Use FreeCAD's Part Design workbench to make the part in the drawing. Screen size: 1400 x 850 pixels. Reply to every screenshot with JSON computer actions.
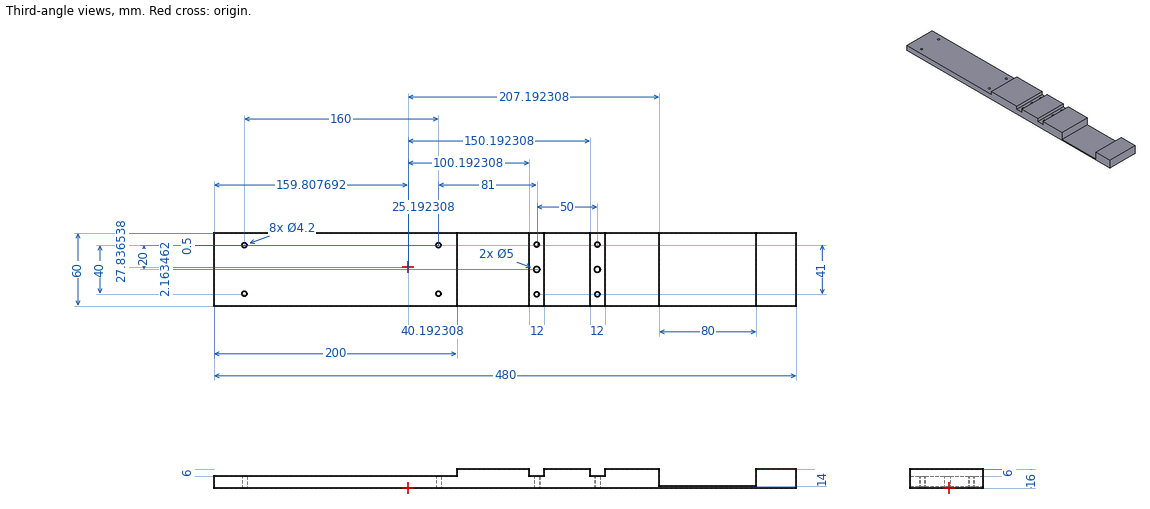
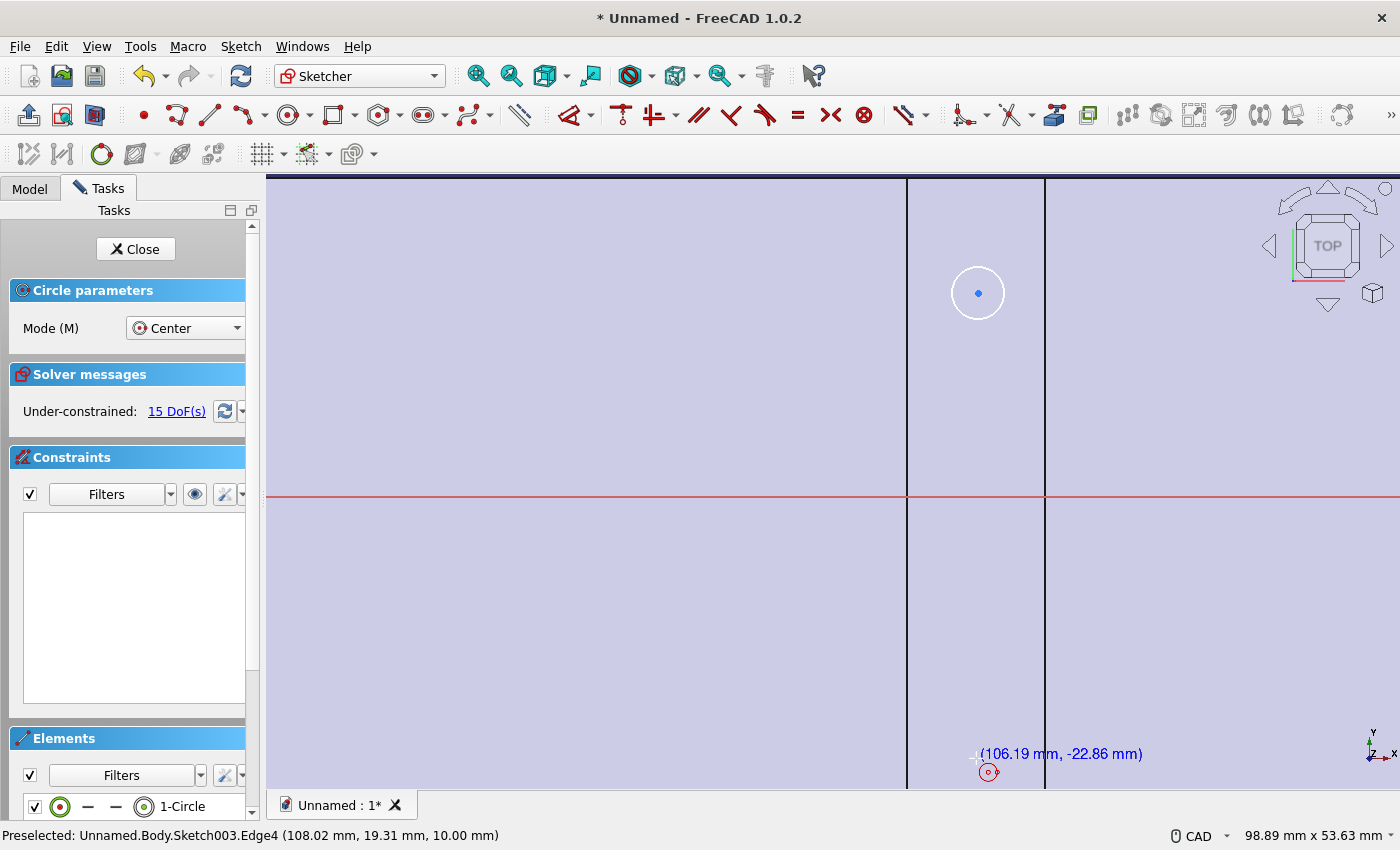
{"action": "scroll", "coordinate": [988, 471], "scroll_direction": "down", "scroll_amount": 8}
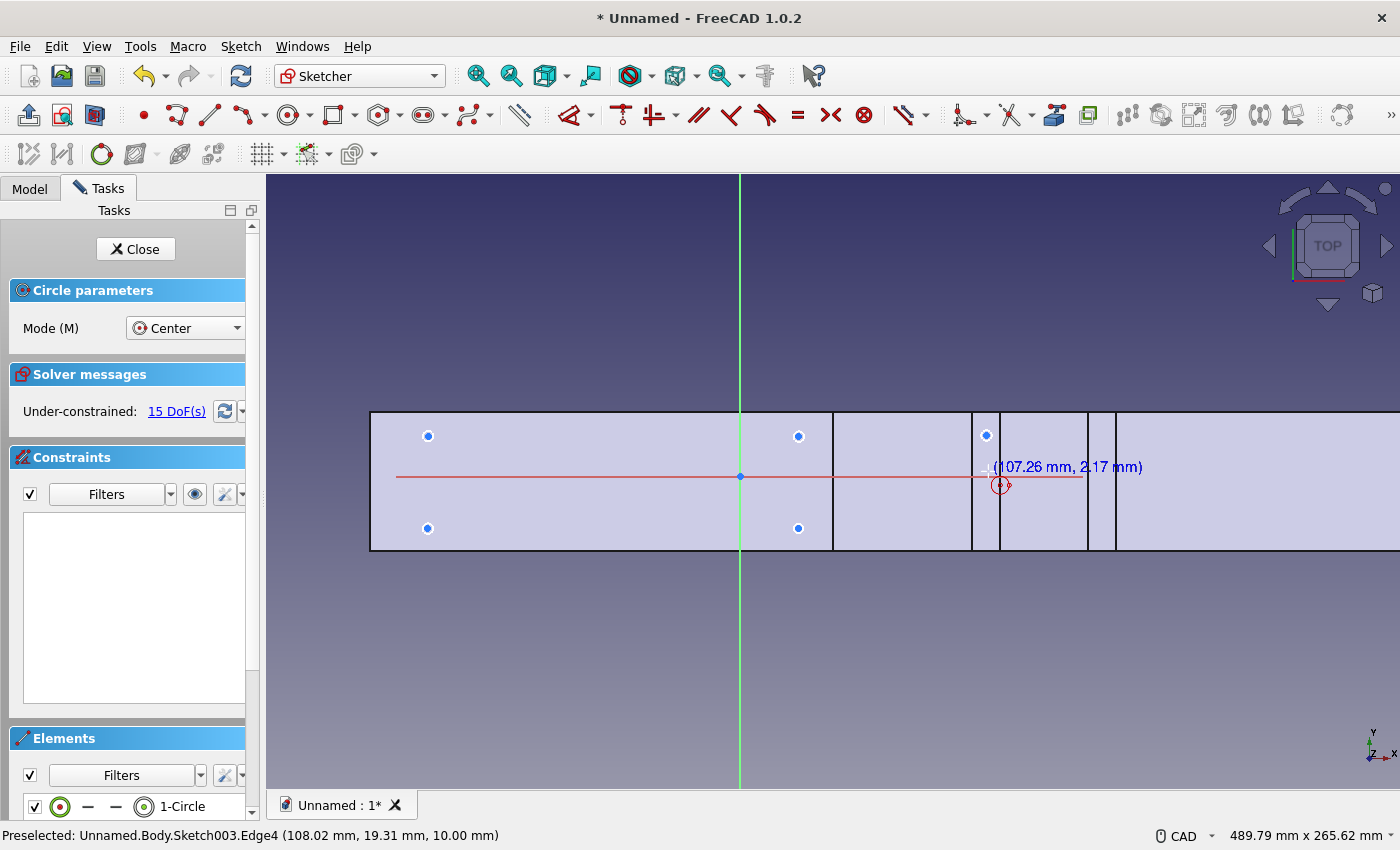
{"action": "left_click", "coordinate": [986, 529]}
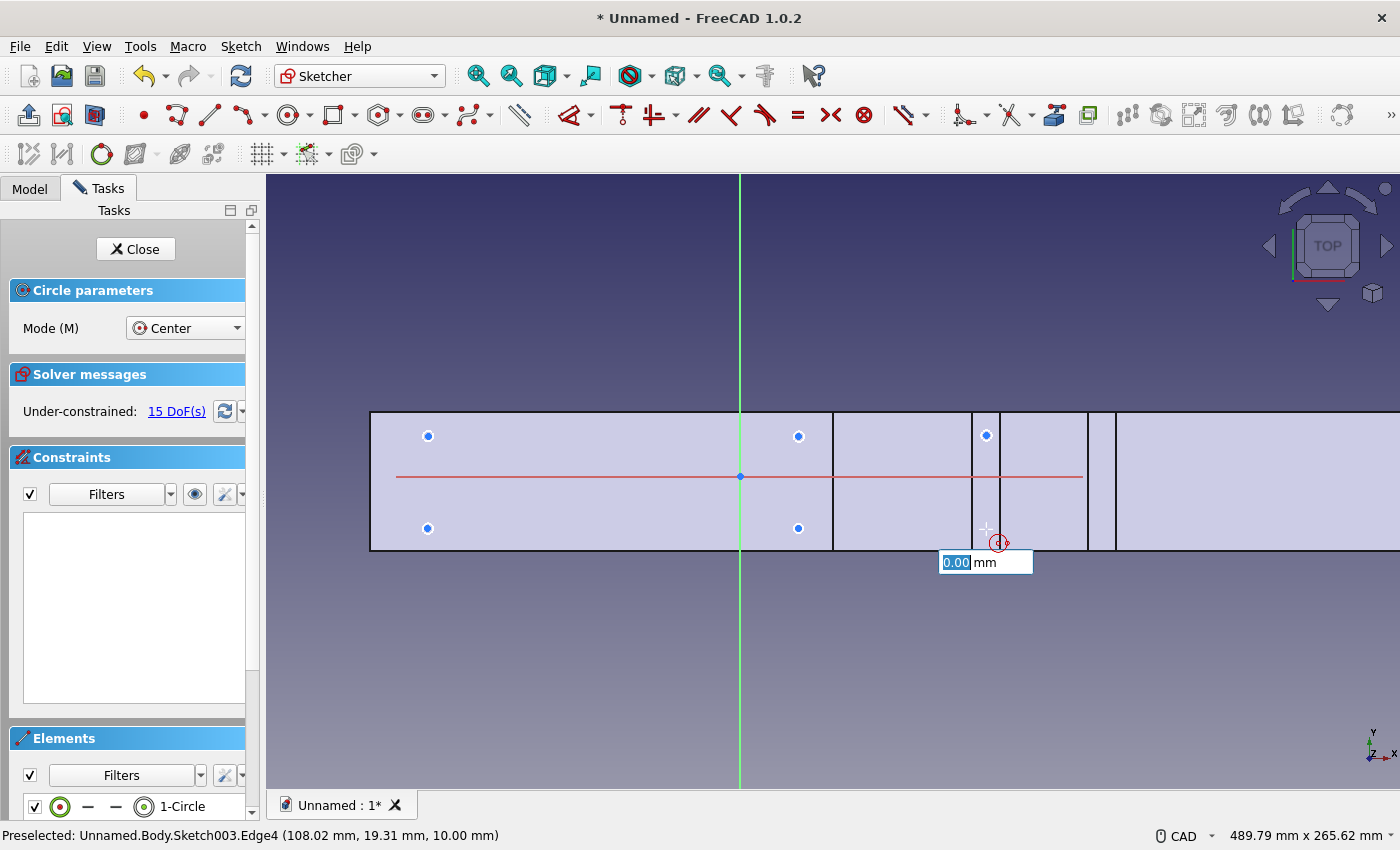
{"action": "scroll", "coordinate": [989, 526], "scroll_direction": "up", "scroll_amount": 6}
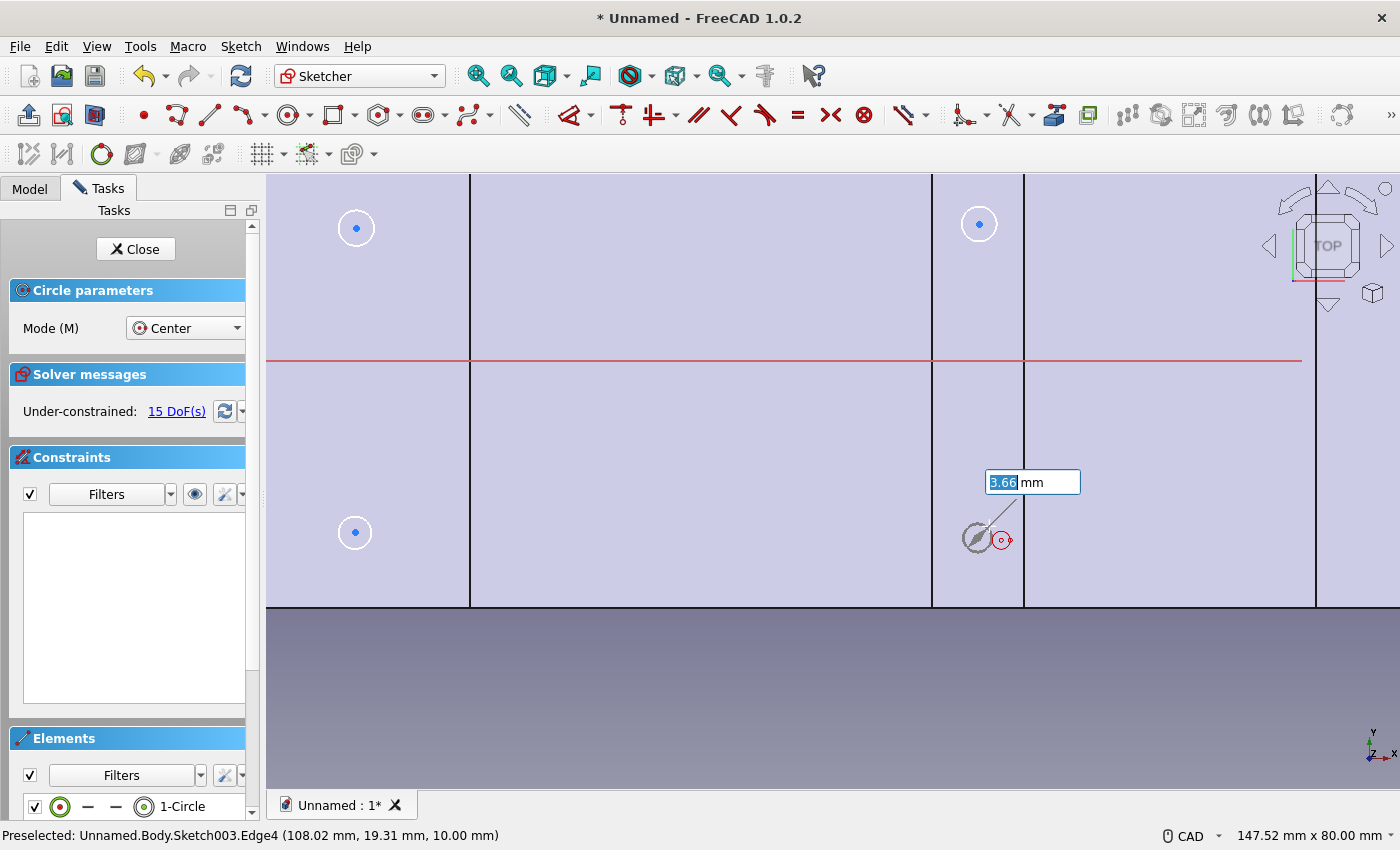
{"action": "left_click", "coordinate": [989, 524]}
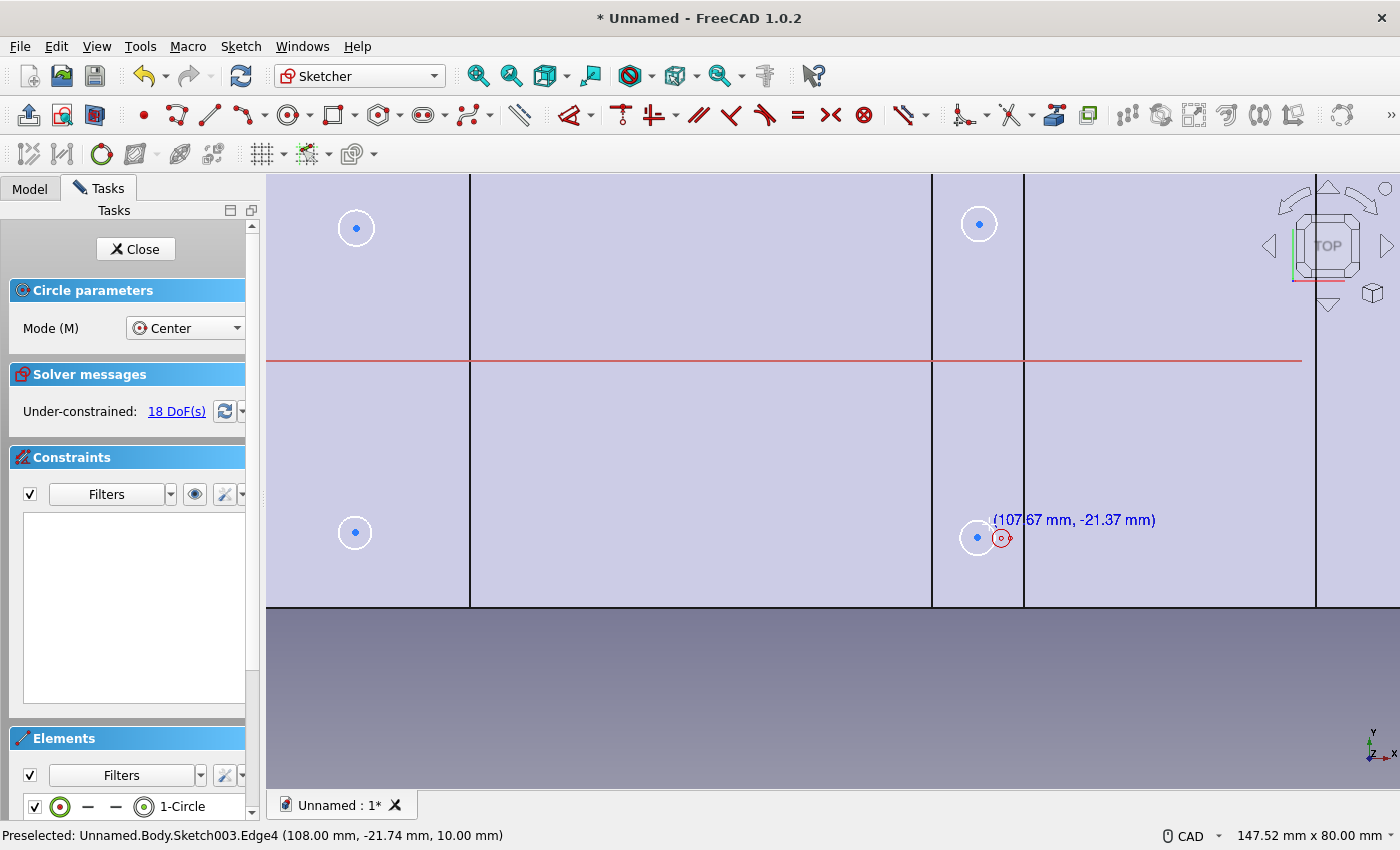
{"action": "scroll", "coordinate": [988, 526], "scroll_direction": "down", "scroll_amount": 6}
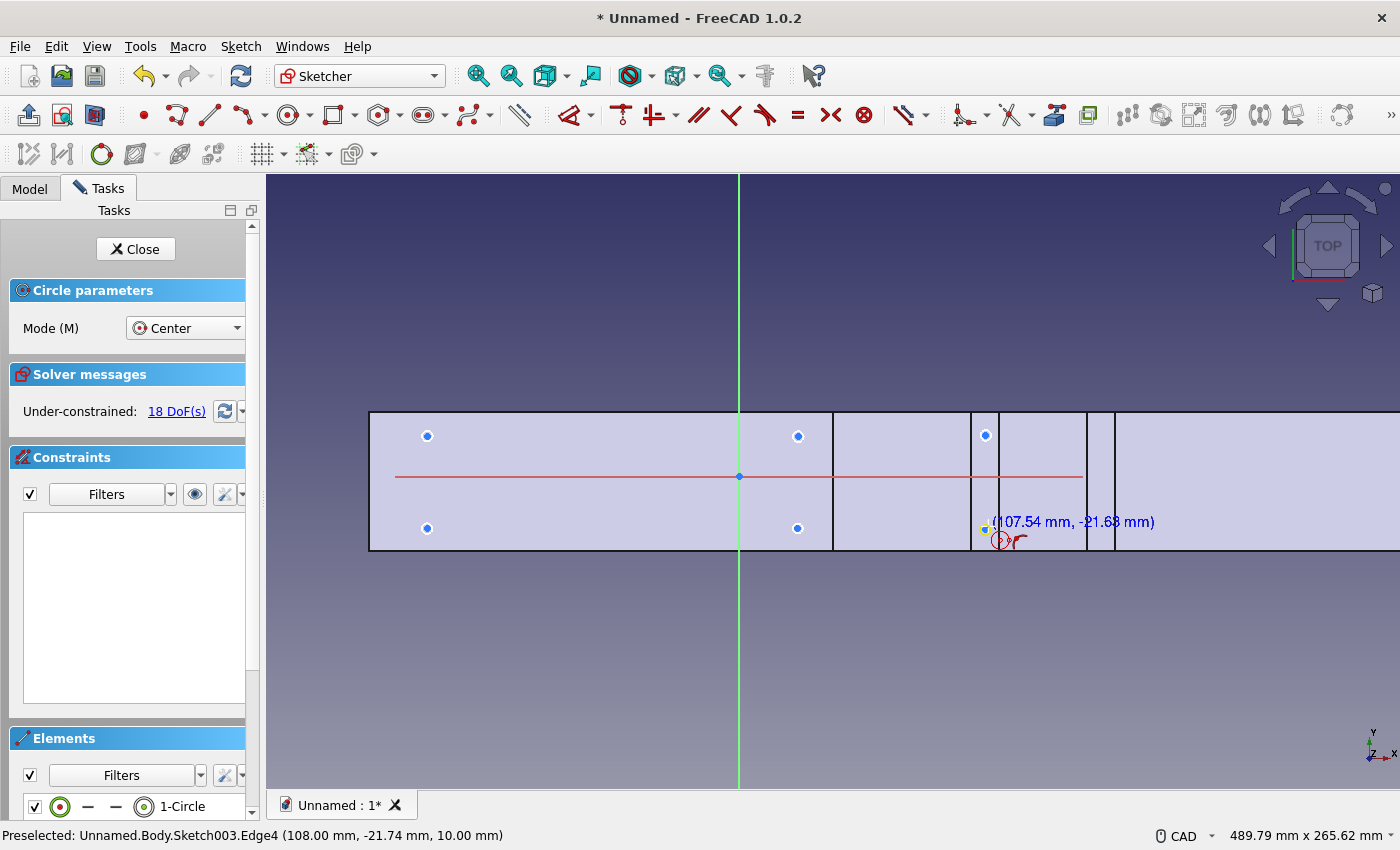
{"action": "scroll", "coordinate": [1101, 434], "scroll_direction": "up", "scroll_amount": 8}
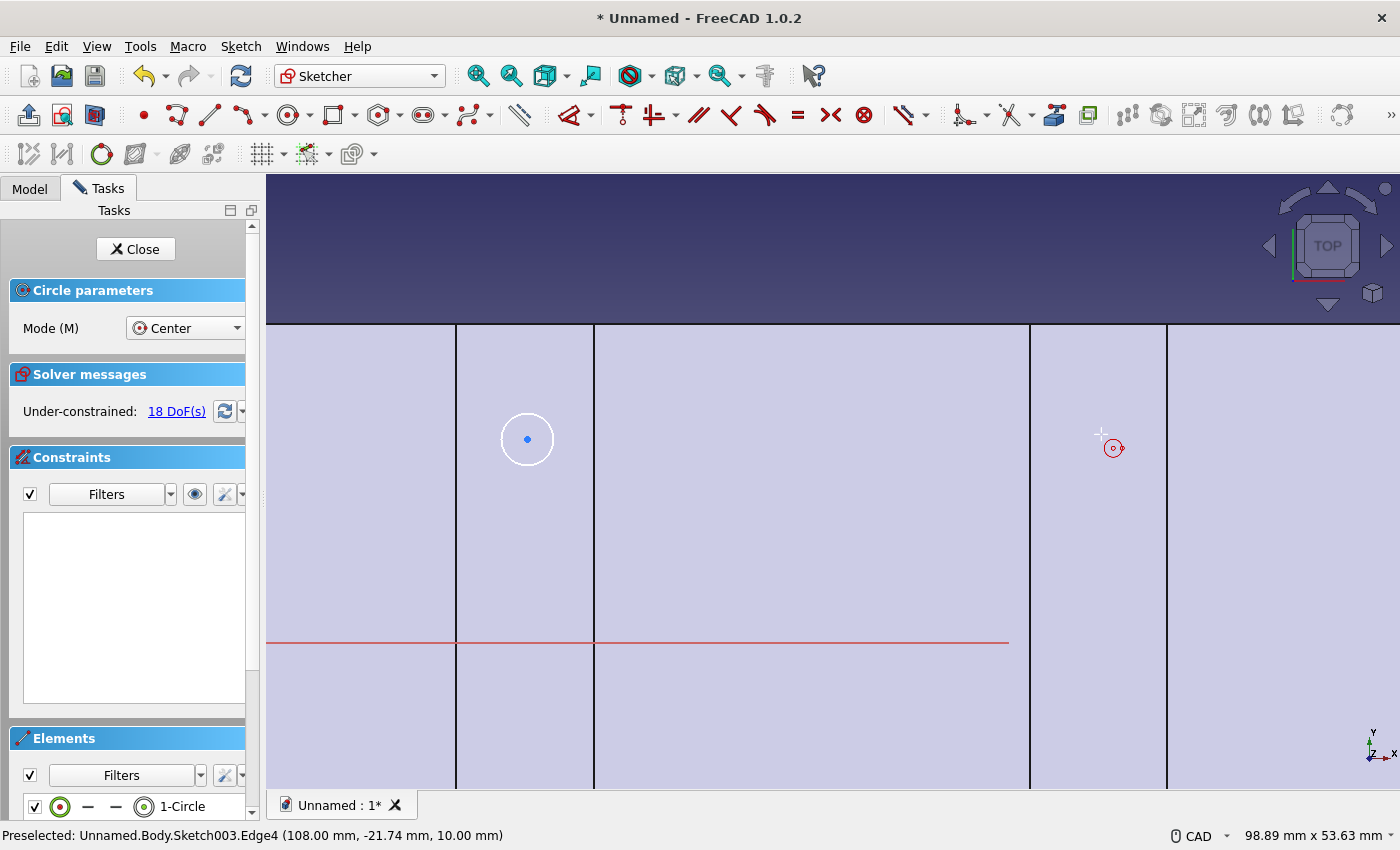
{"action": "scroll", "coordinate": [1102, 434], "scroll_direction": "down", "scroll_amount": 8}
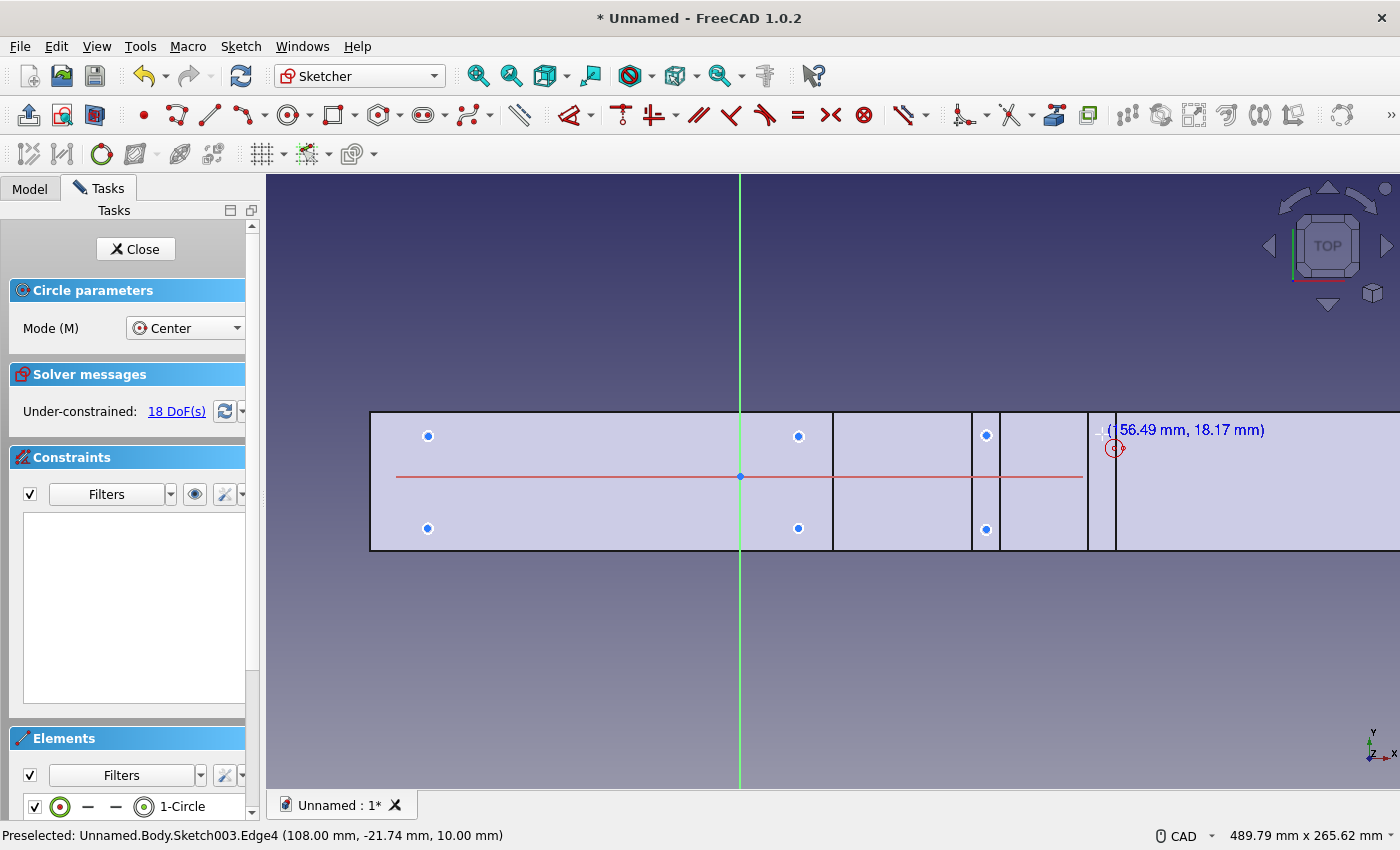
{"action": "left_click", "coordinate": [1102, 434]}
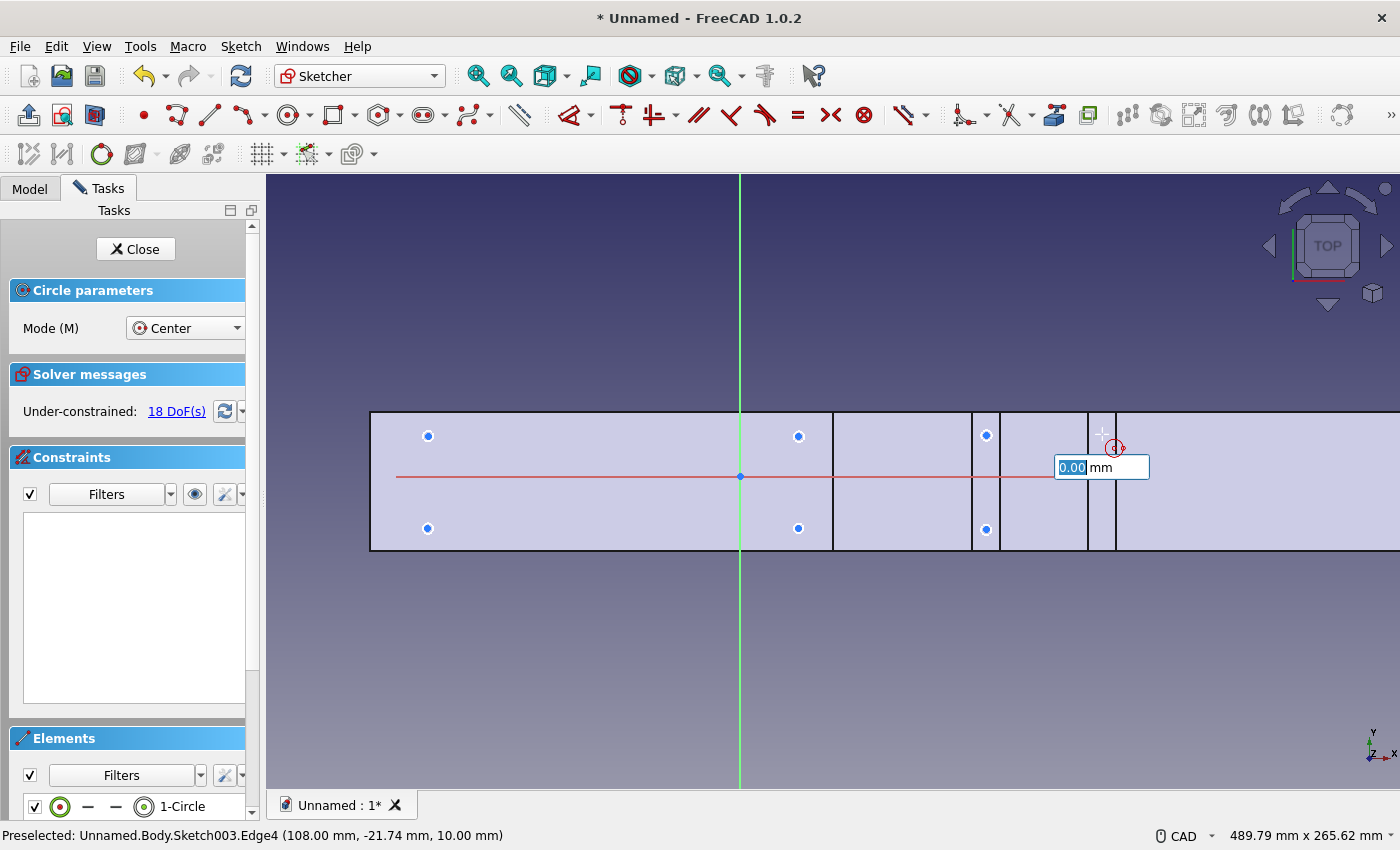
{"action": "scroll", "coordinate": [1105, 431], "scroll_direction": "up", "scroll_amount": 6}